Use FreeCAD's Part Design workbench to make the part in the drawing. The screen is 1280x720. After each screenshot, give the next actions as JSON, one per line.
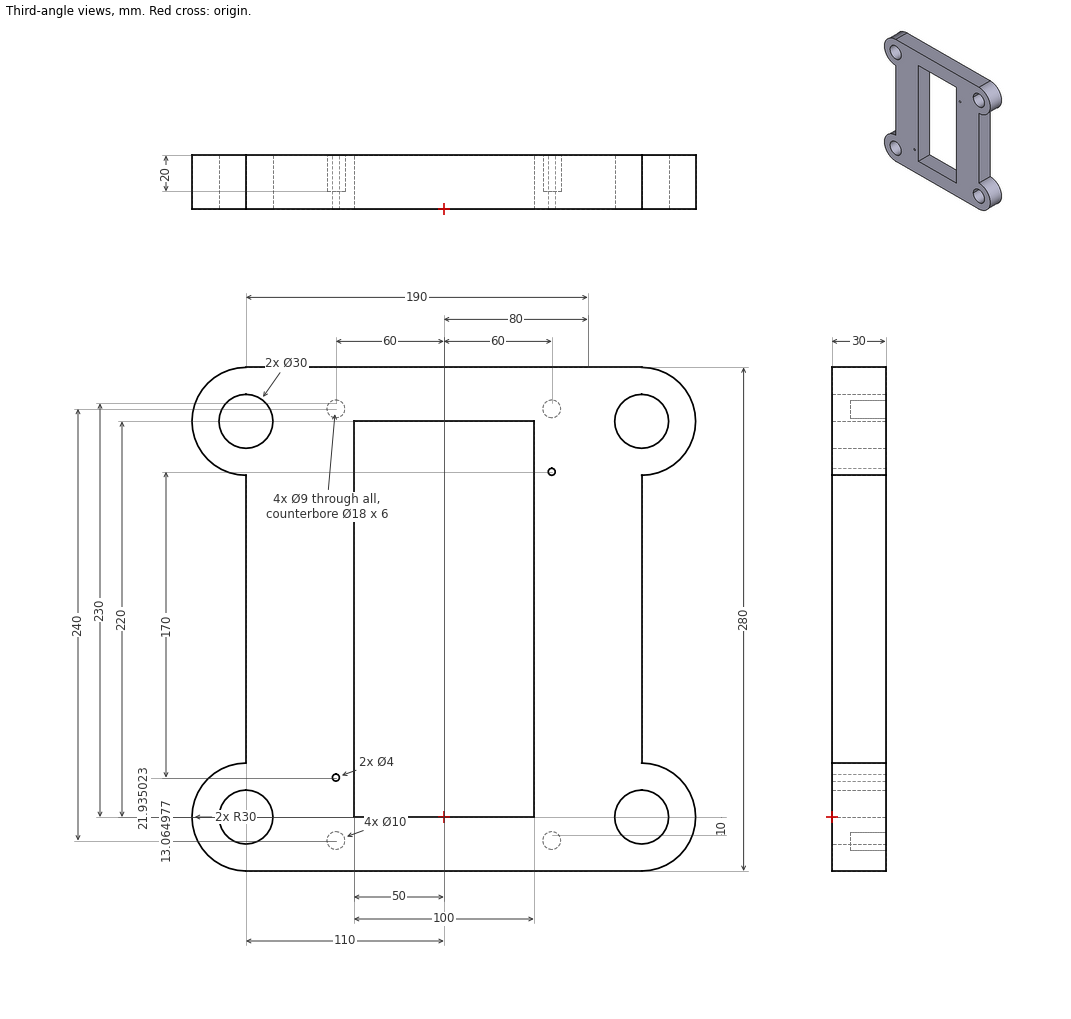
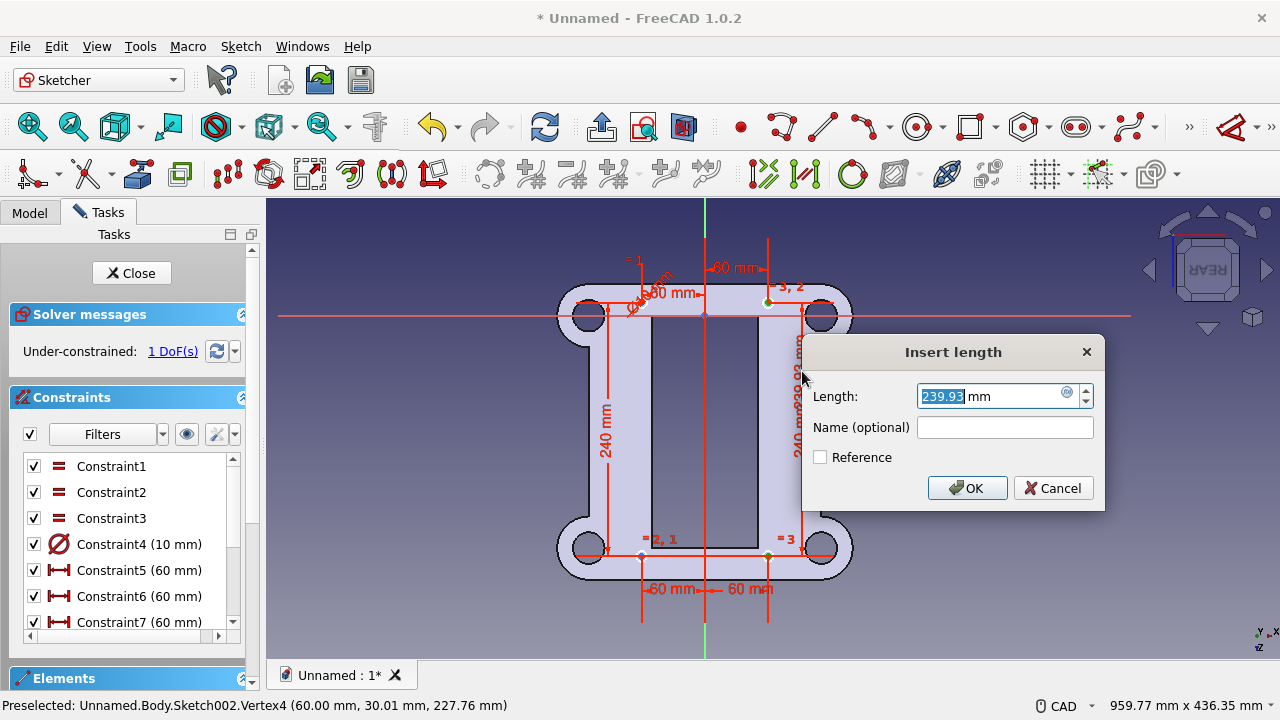
{"action": "type", "text": "240"}
{"action": "key", "text": "Return"}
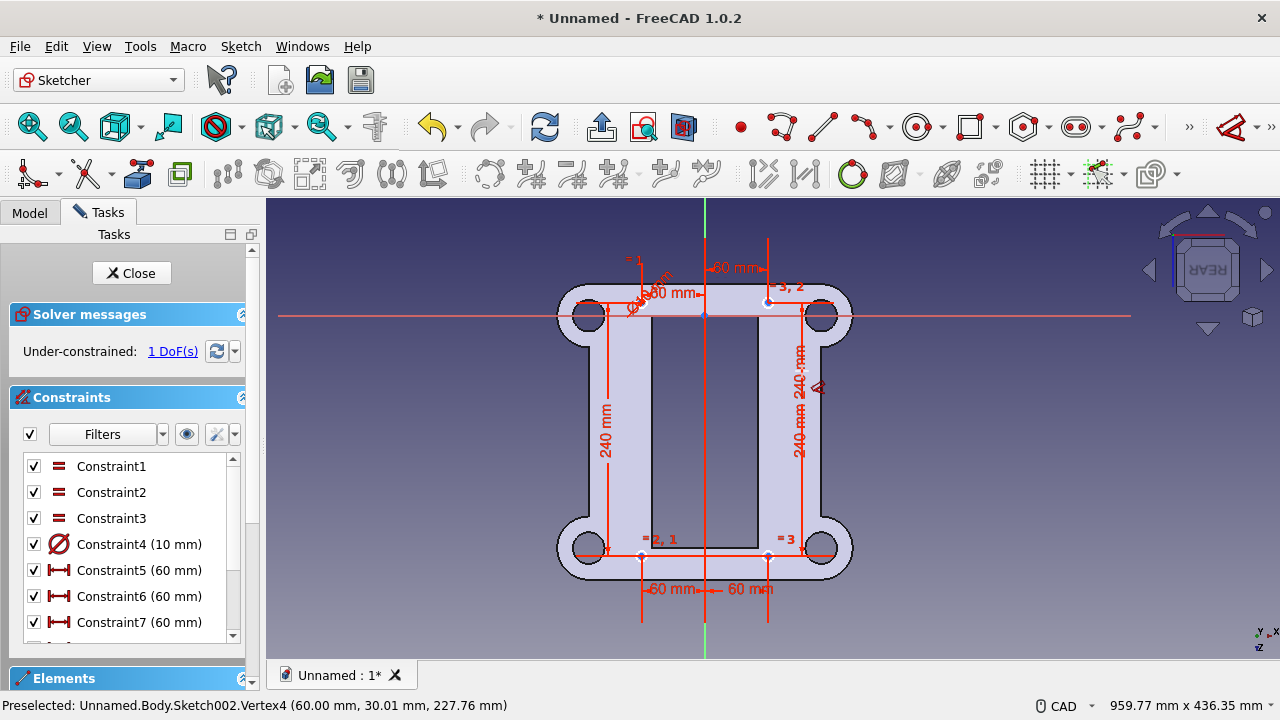
{"action": "scroll", "coordinate": [642, 303], "scroll_direction": "up", "scroll_amount": 6}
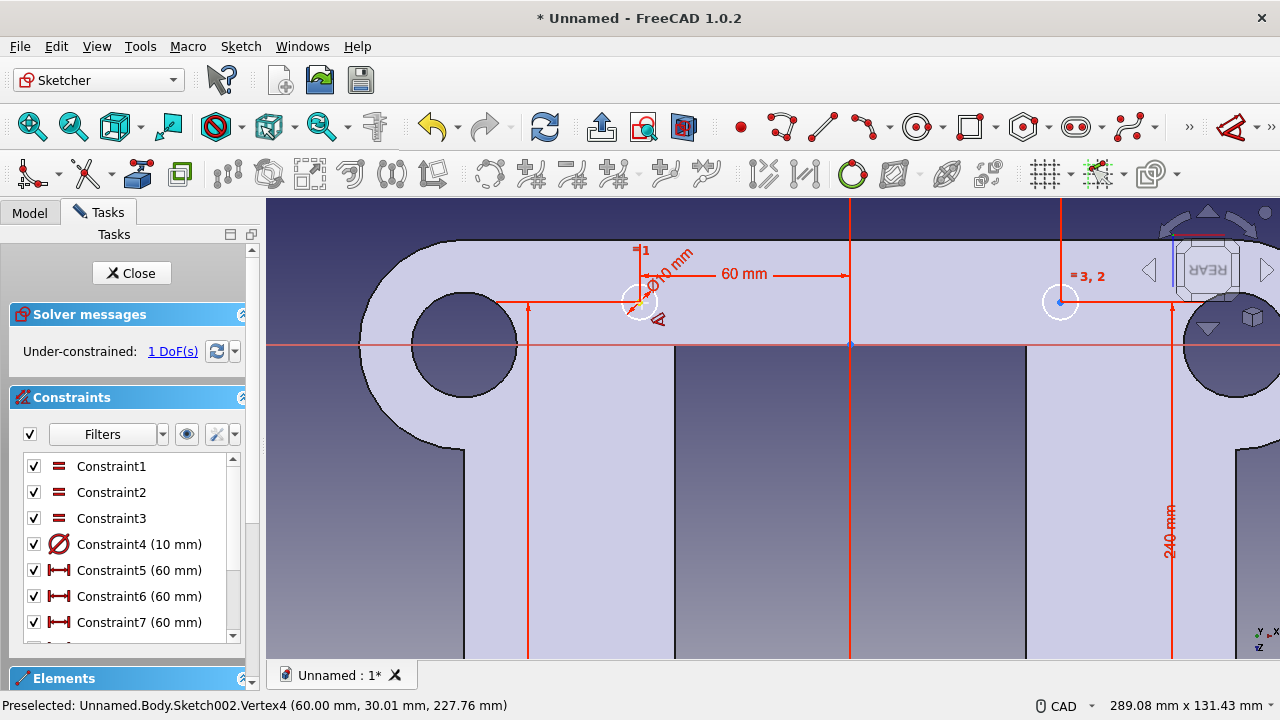
{"action": "left_click", "coordinate": [640, 302]}
{"action": "left_click", "coordinate": [606, 323]}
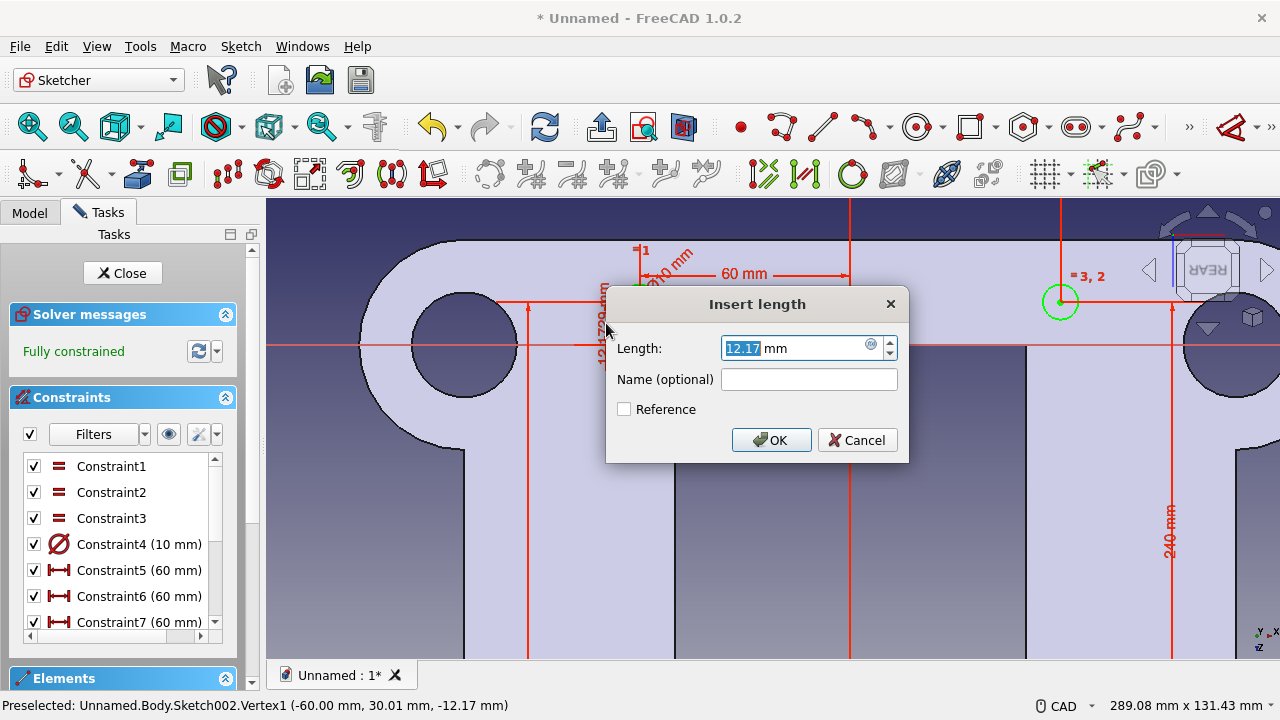
{"action": "type", "text": "13.064977"}
{"action": "key", "text": "Return"}
{"action": "key", "text": "Escape"}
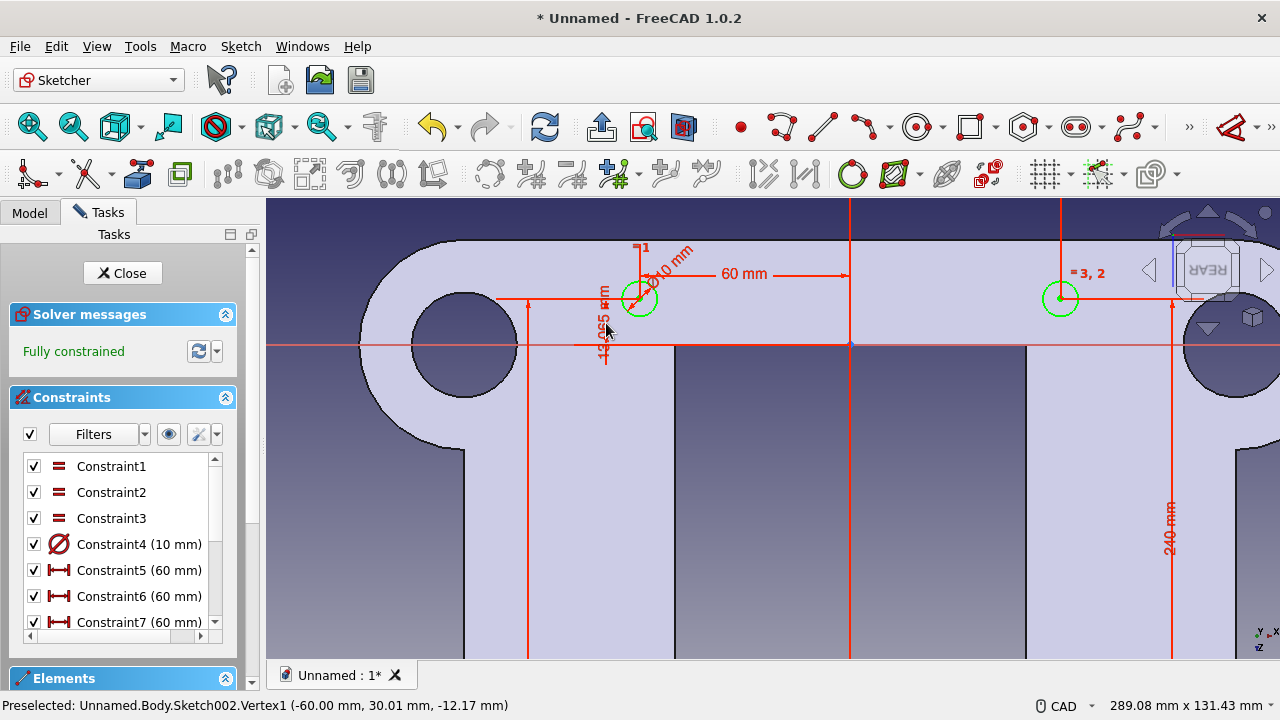
{"action": "left_click", "coordinate": [123, 273]}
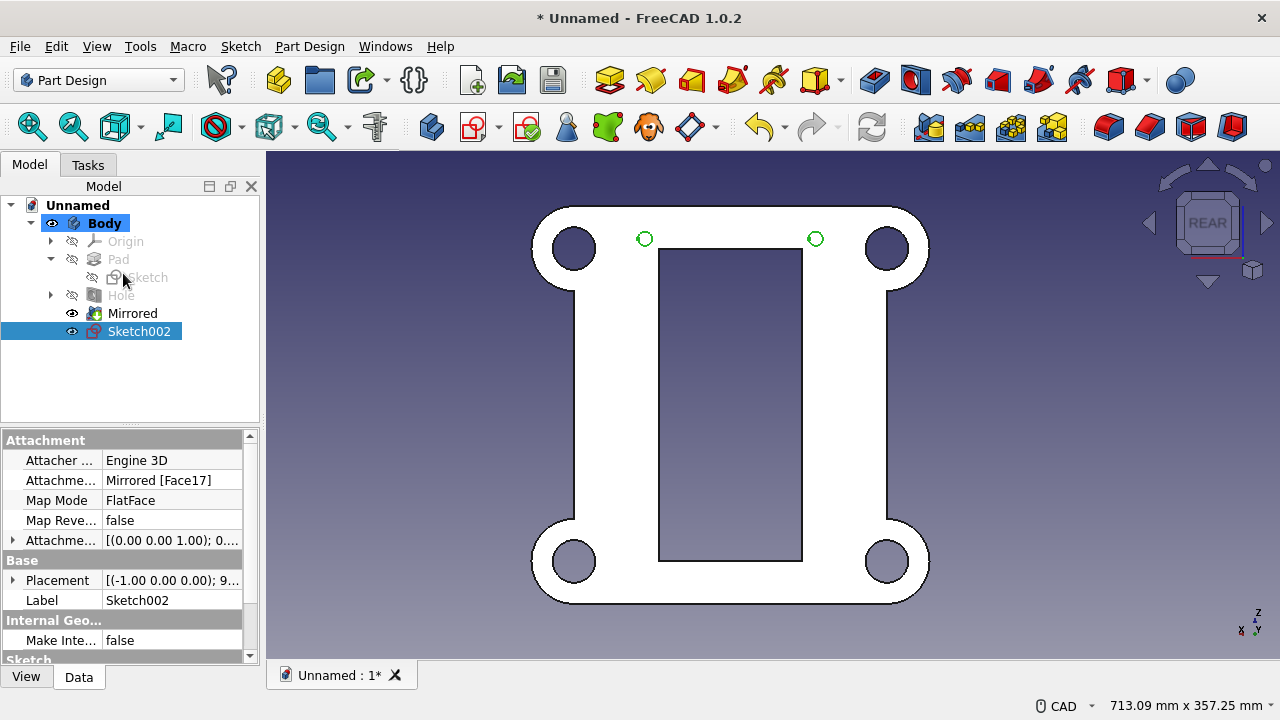
{"action": "left_click", "coordinate": [875, 80]}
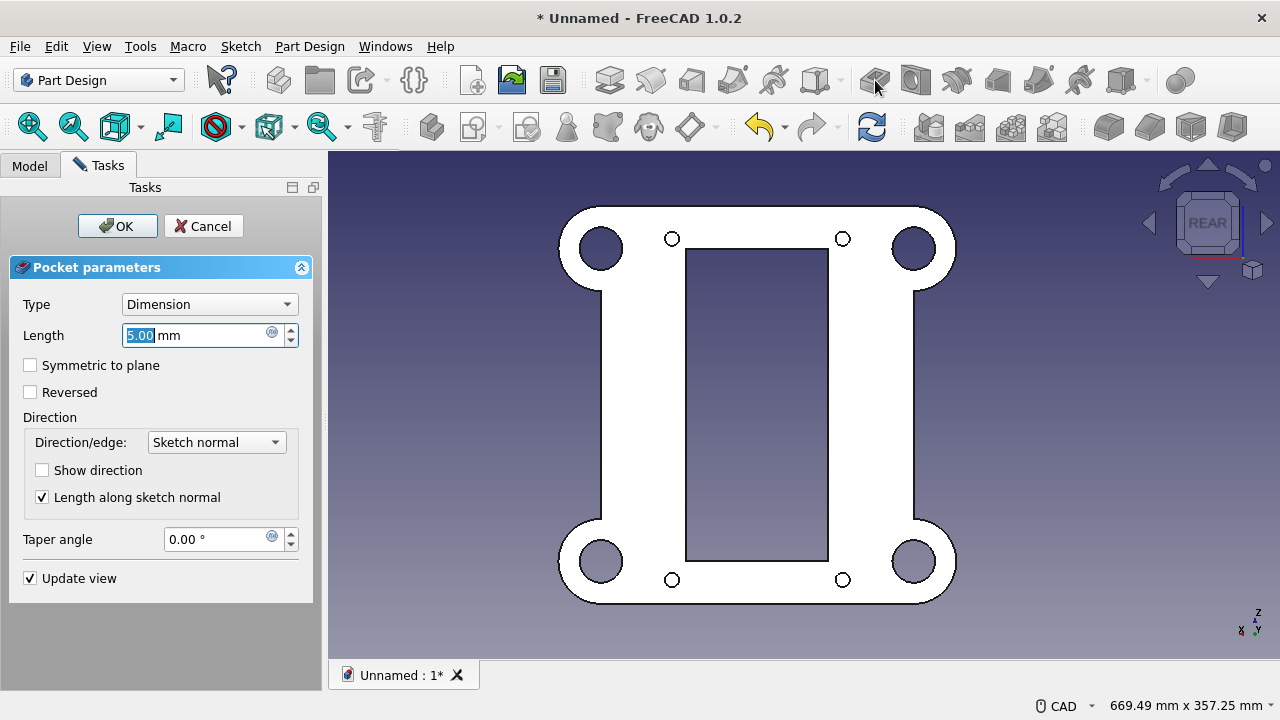
{"action": "type", "text": "20"}
{"action": "key", "text": "Tab"}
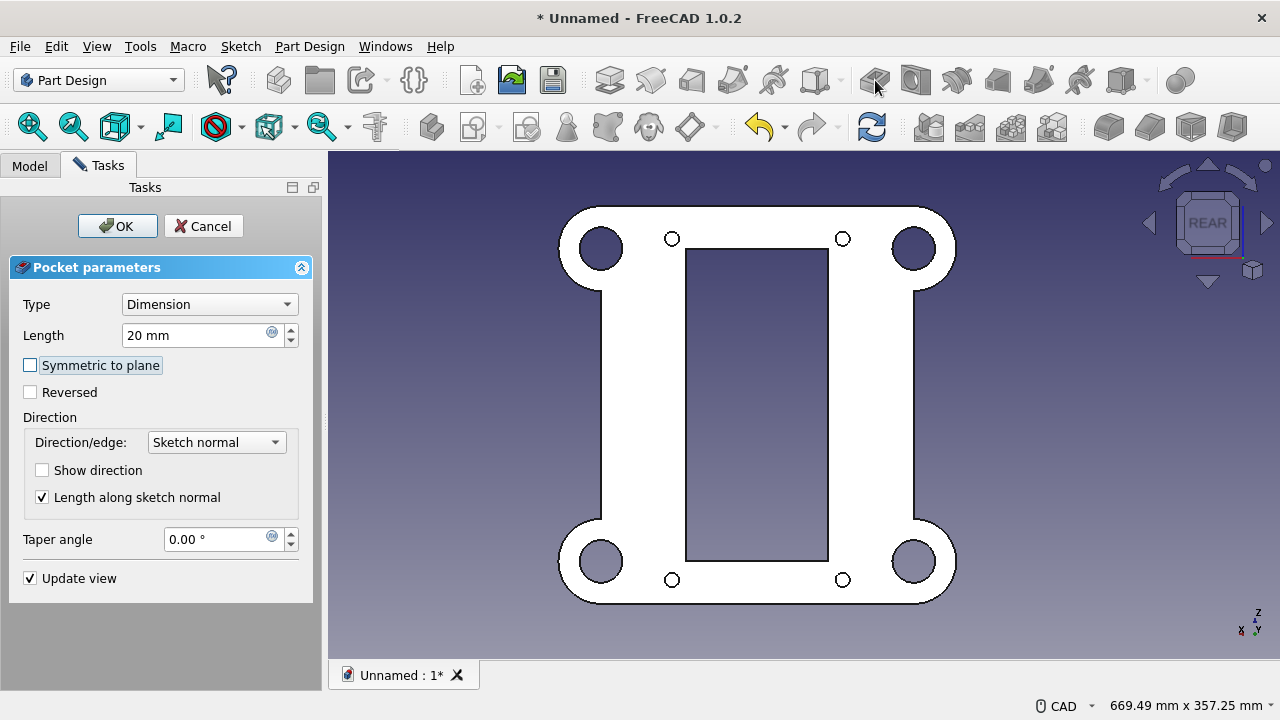
{"action": "left_click", "coordinate": [118, 226]}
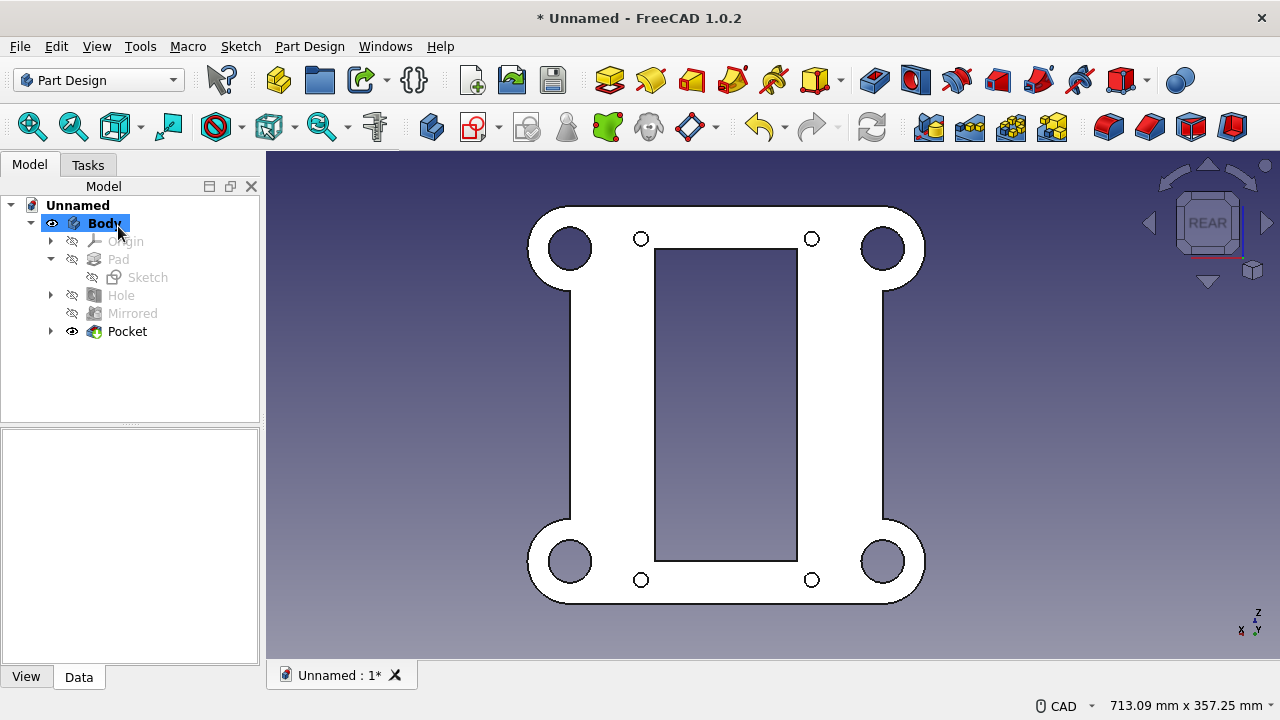
{"action": "left_click", "coordinate": [840, 347]}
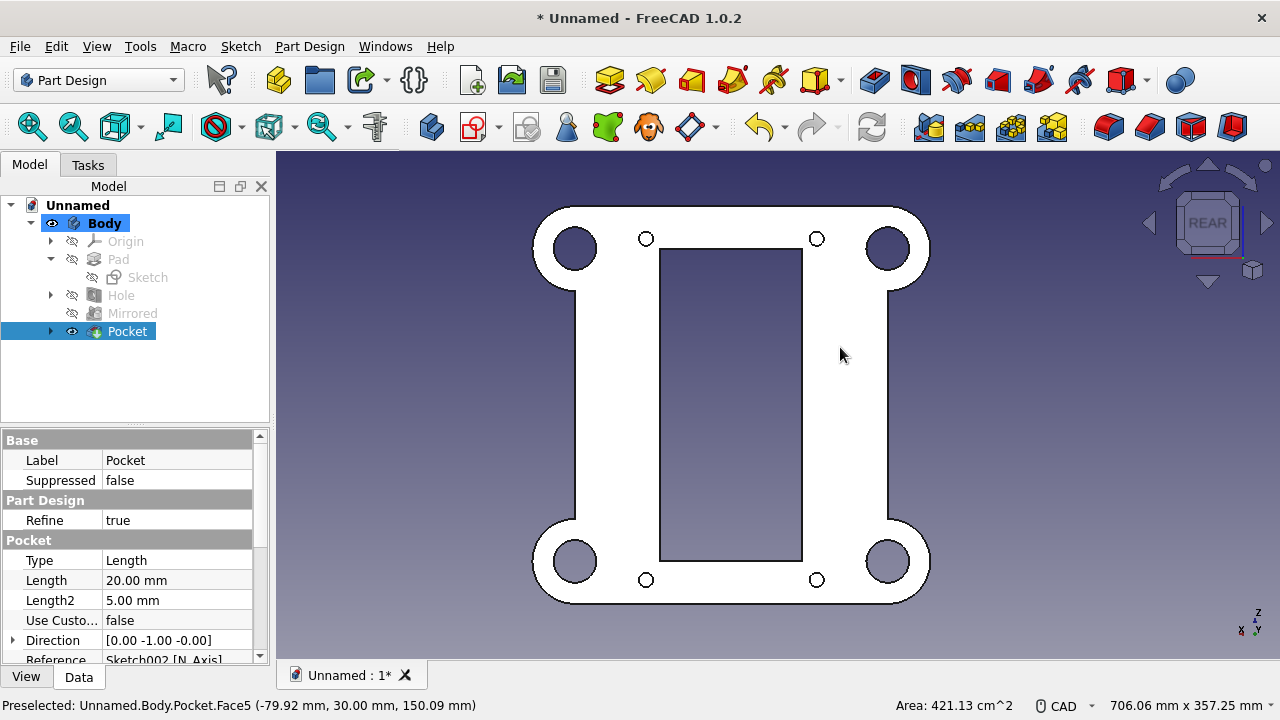
{"action": "left_click", "coordinate": [472, 128]}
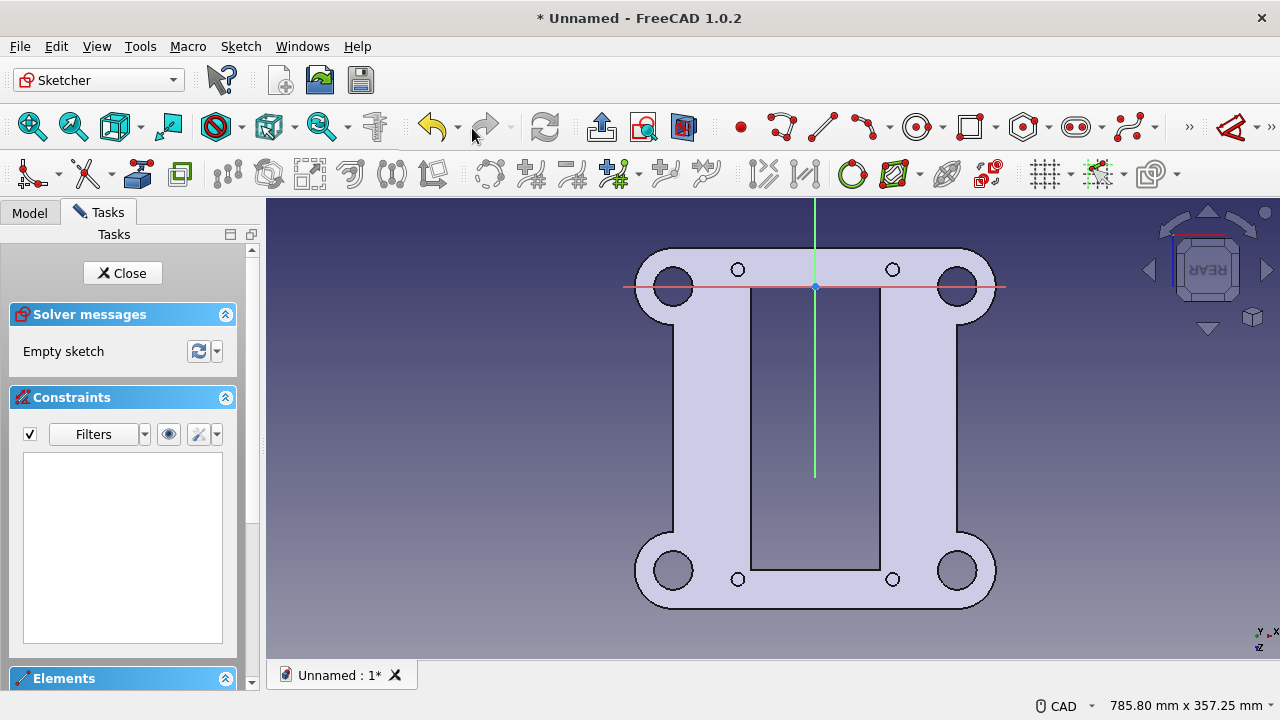
{"action": "key", "text": "g c"}